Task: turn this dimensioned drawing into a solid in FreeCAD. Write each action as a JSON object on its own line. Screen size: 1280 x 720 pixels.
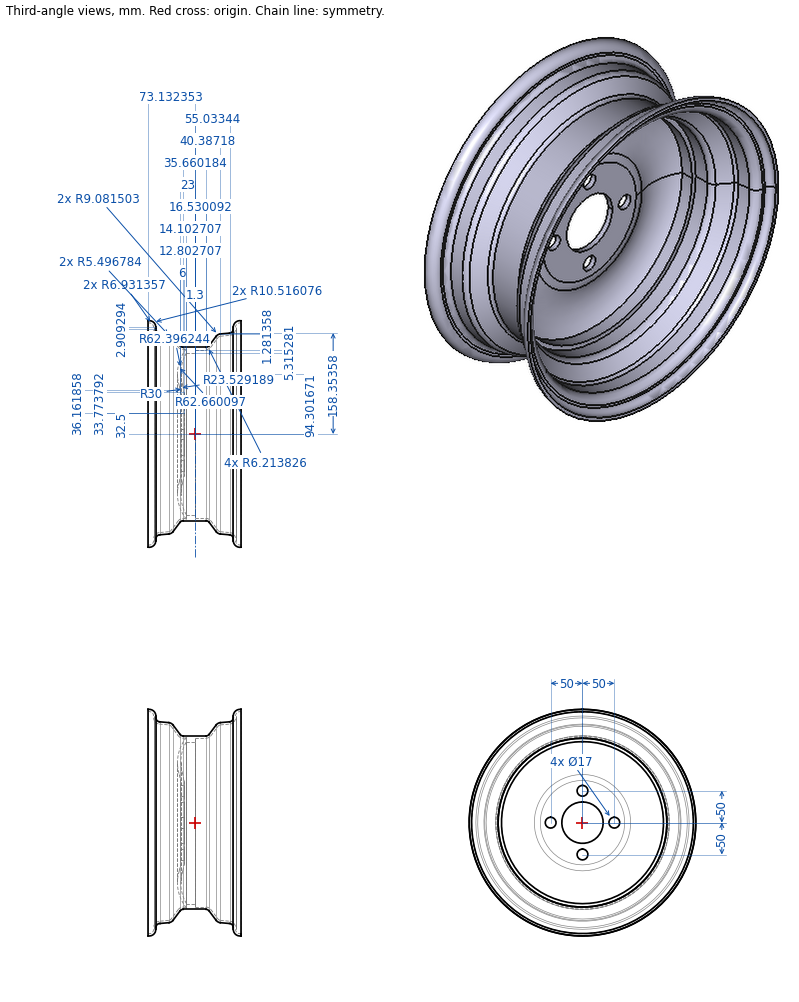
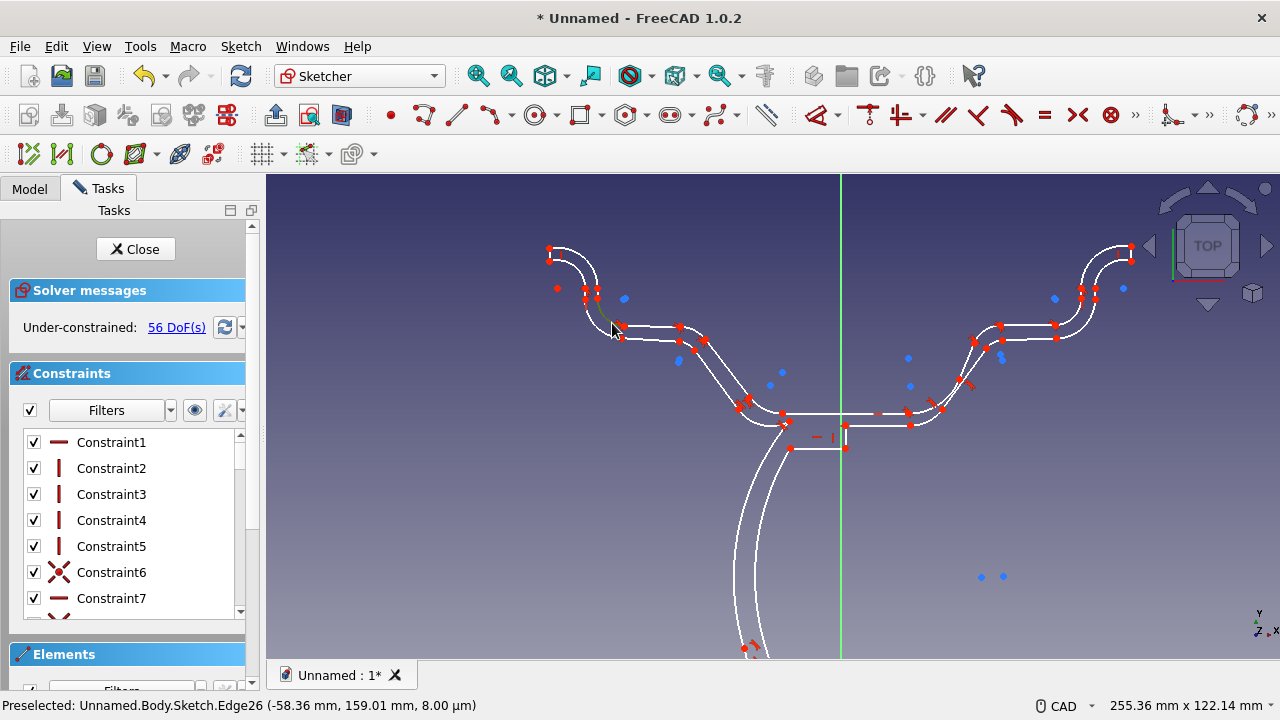
{"action": "left_click", "coordinate": [589, 316]}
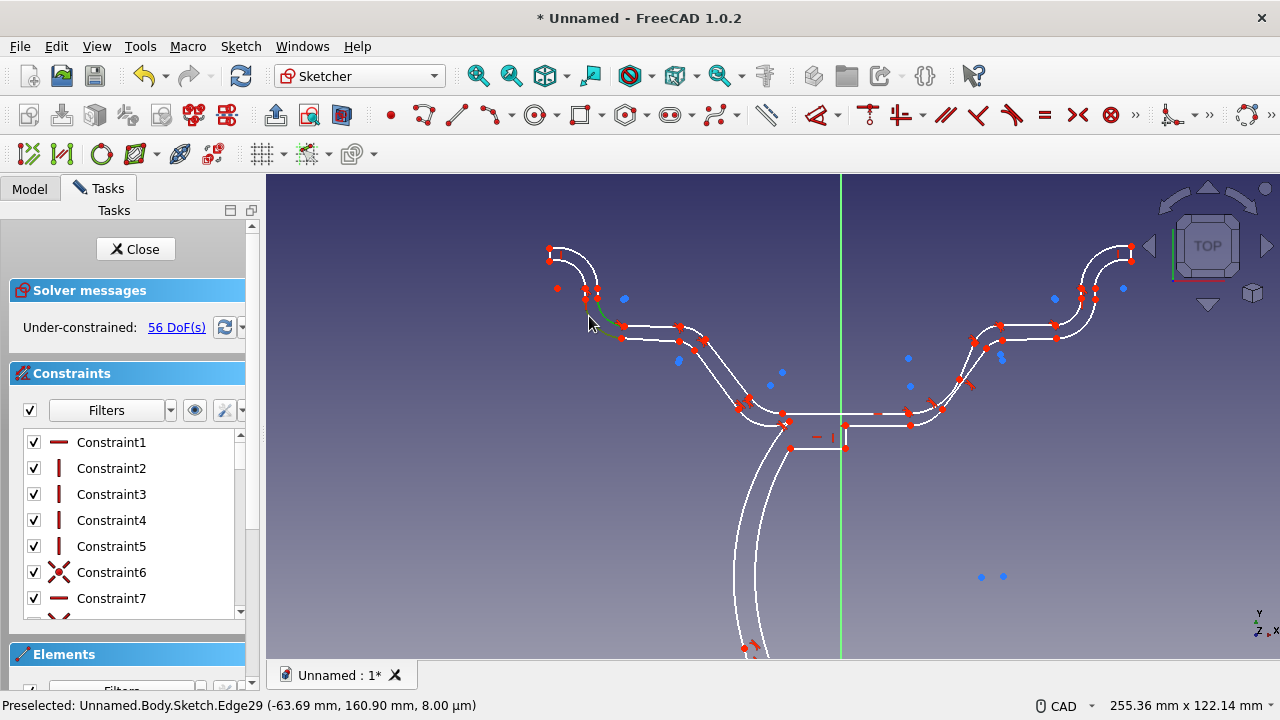
{"action": "left_click", "coordinate": [868, 116]}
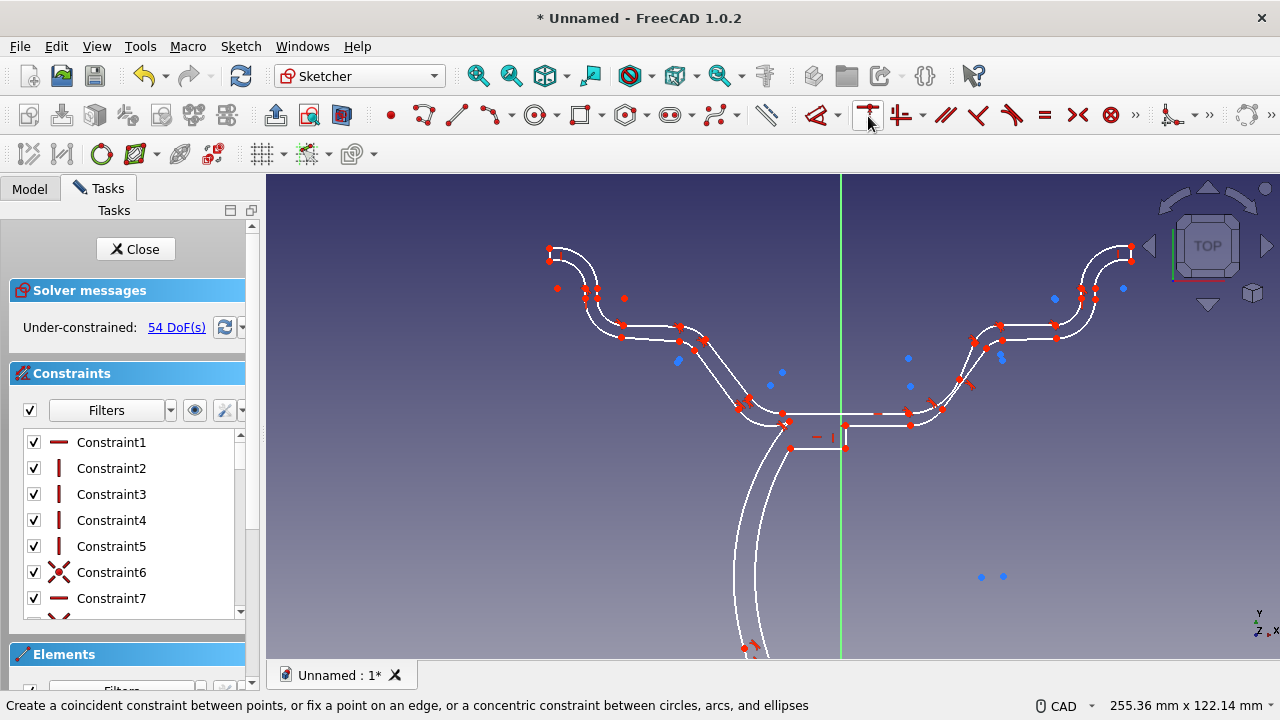
{"action": "left_click", "coordinate": [695, 330]}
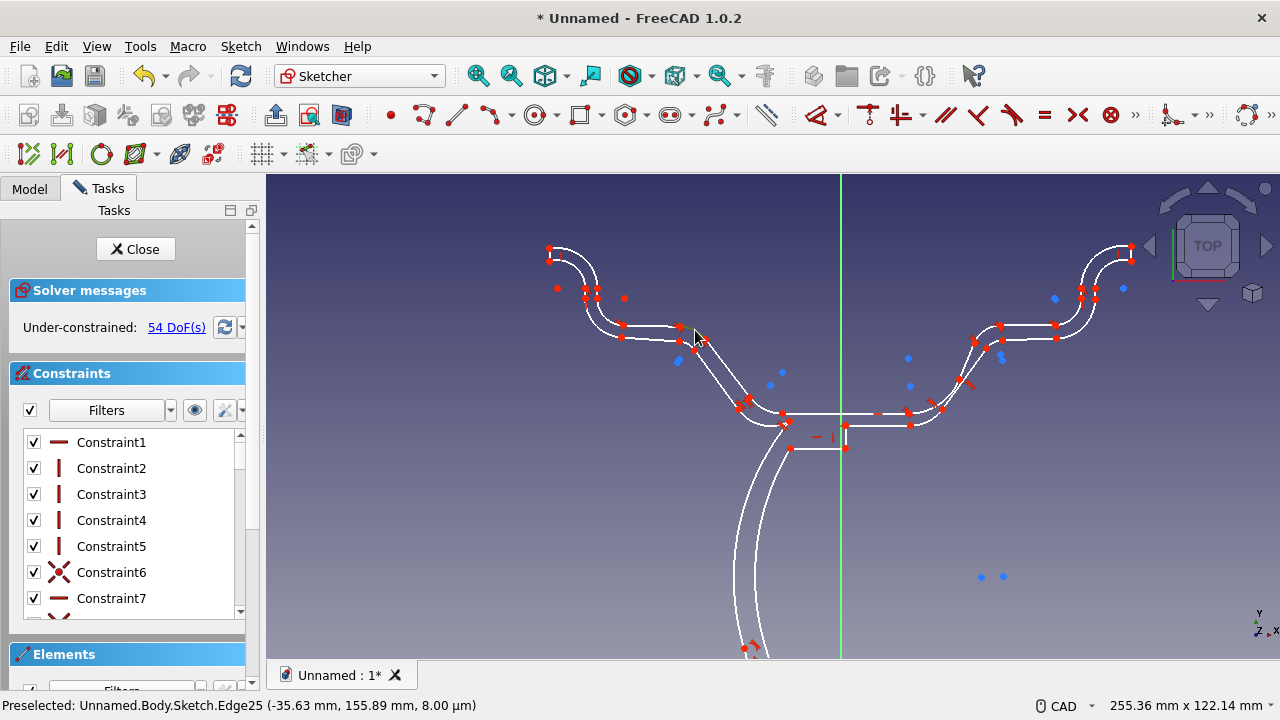
{"action": "scroll", "coordinate": [688, 344], "scroll_direction": "up", "scroll_amount": 3}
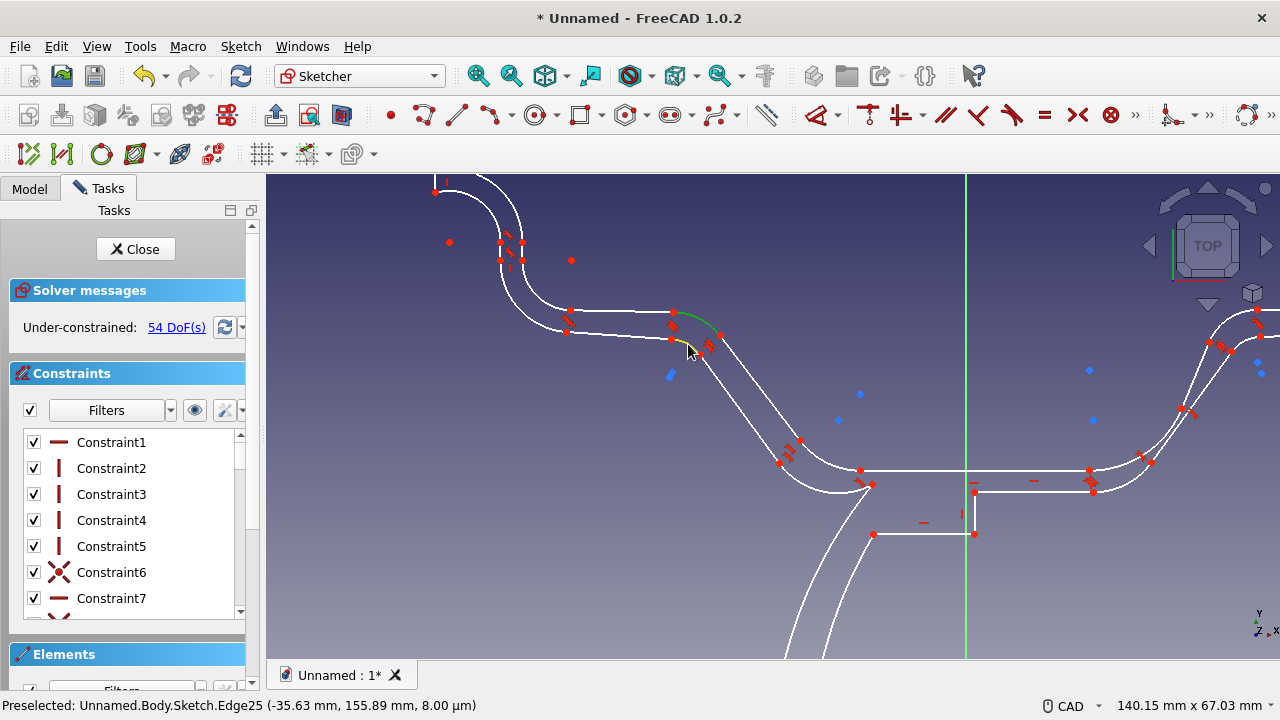
{"action": "left_click", "coordinate": [688, 344]}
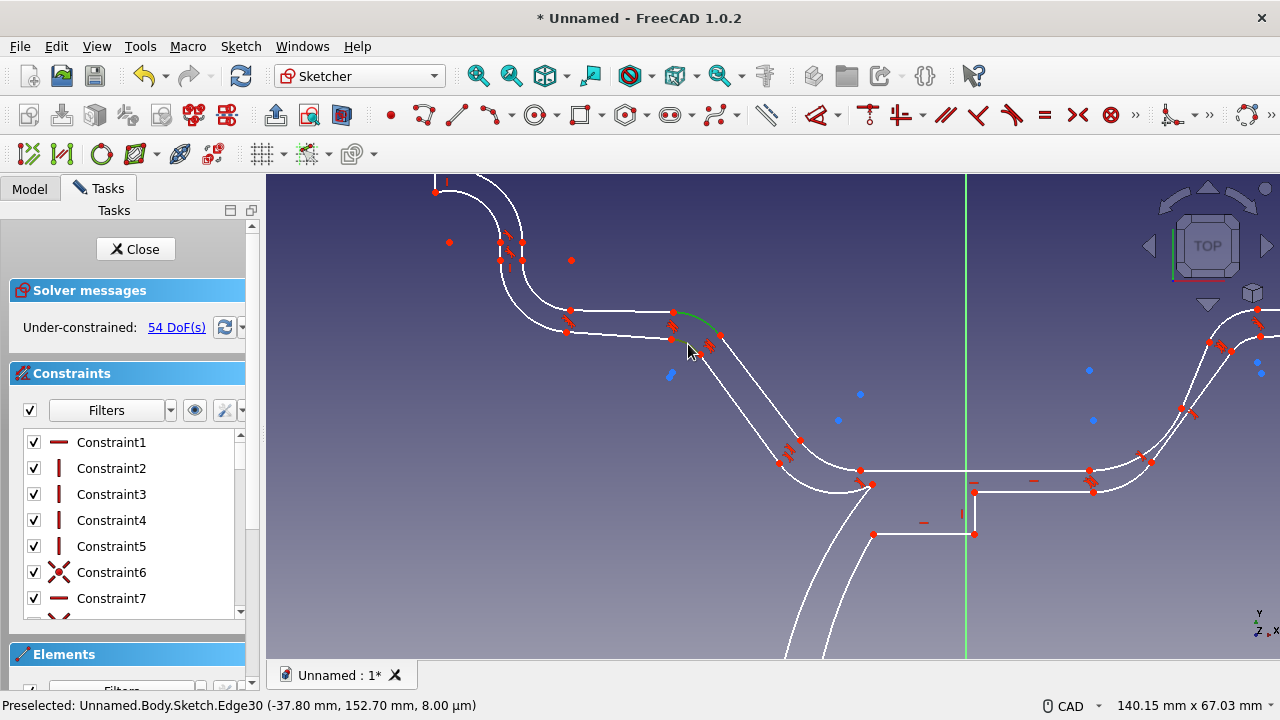
{"action": "key", "text": "c"}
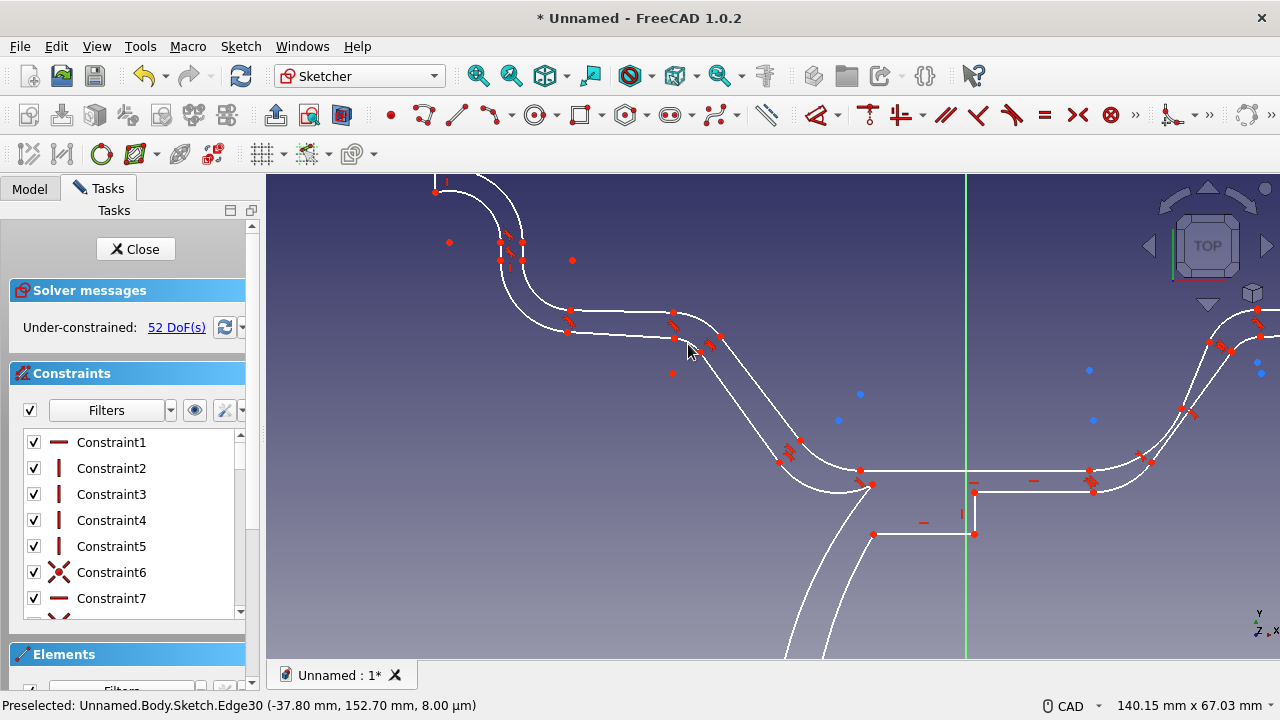
{"action": "left_click", "coordinate": [815, 456]}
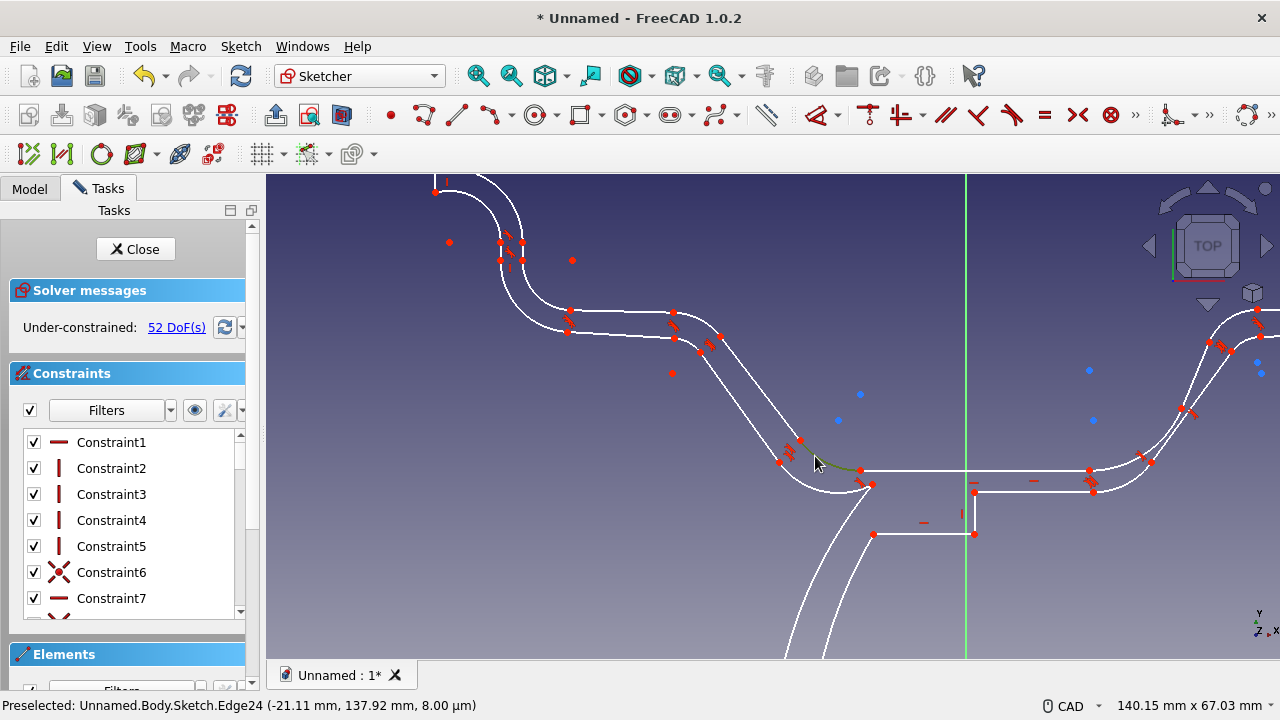
{"action": "left_click", "coordinate": [802, 484]}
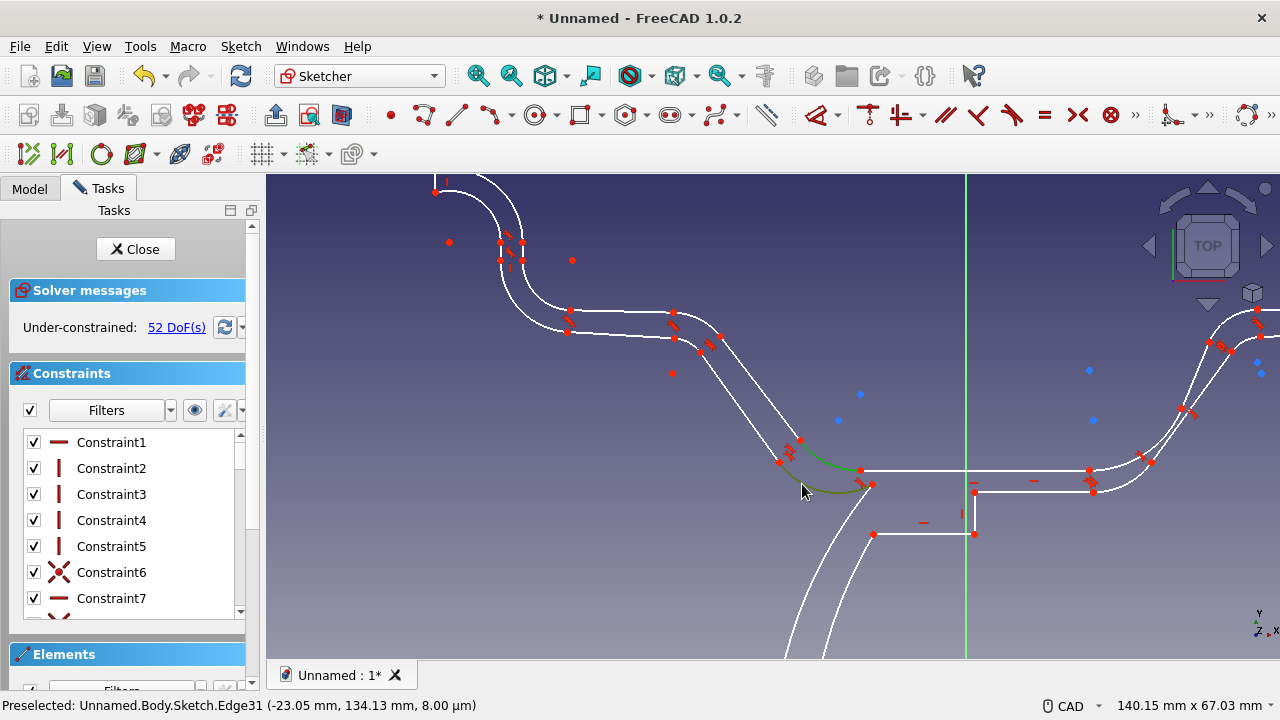
{"action": "key", "text": "c"}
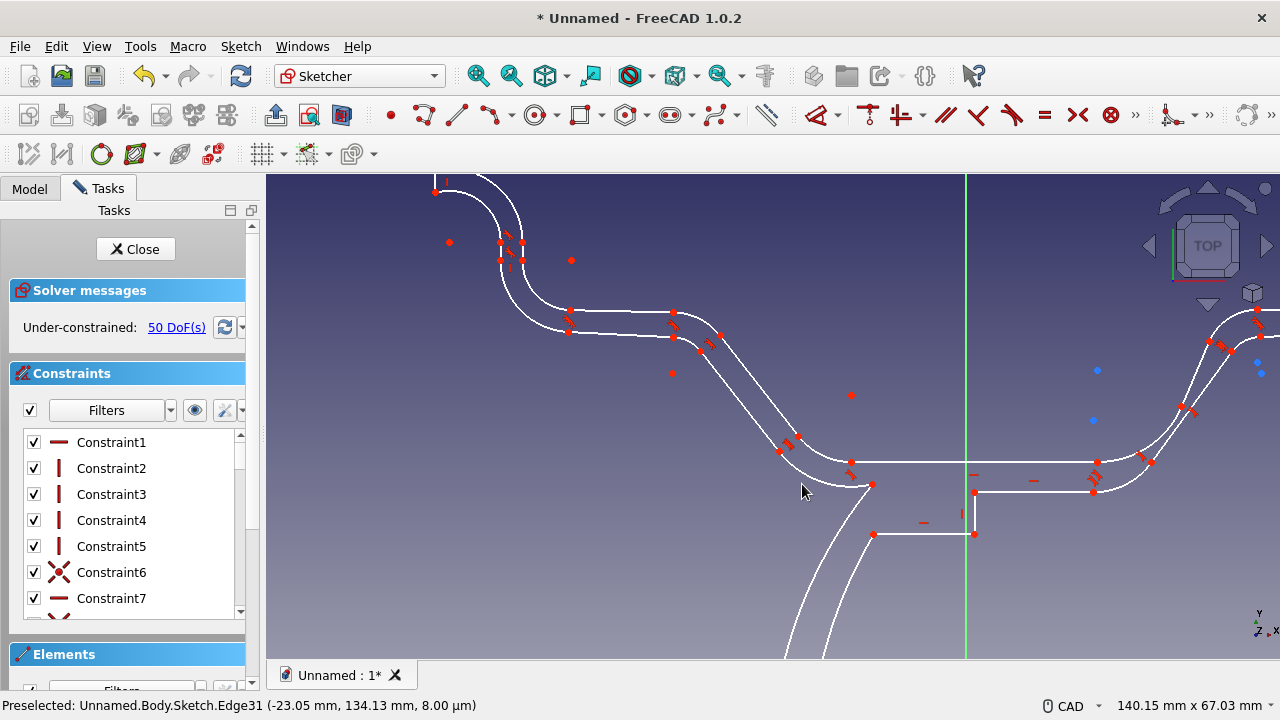
{"action": "scroll", "coordinate": [619, 288], "scroll_direction": "down", "scroll_amount": 7}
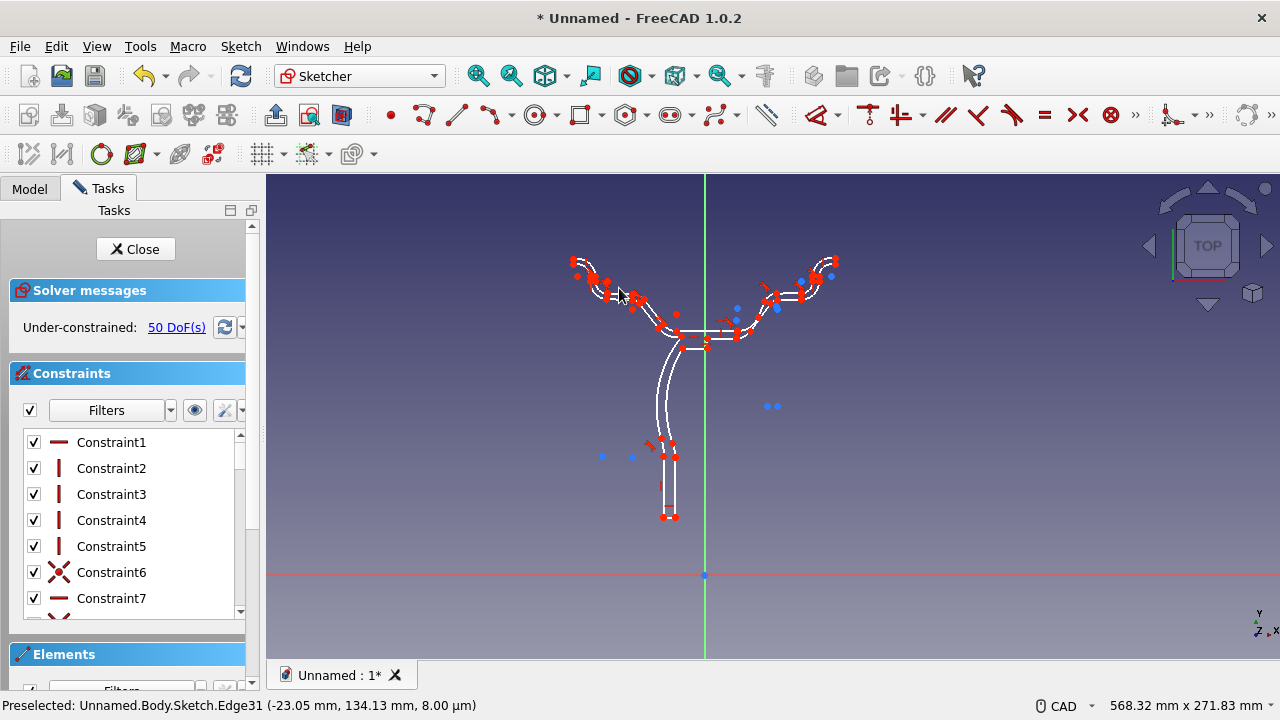
{"action": "scroll", "coordinate": [745, 330], "scroll_direction": "up", "scroll_amount": 5}